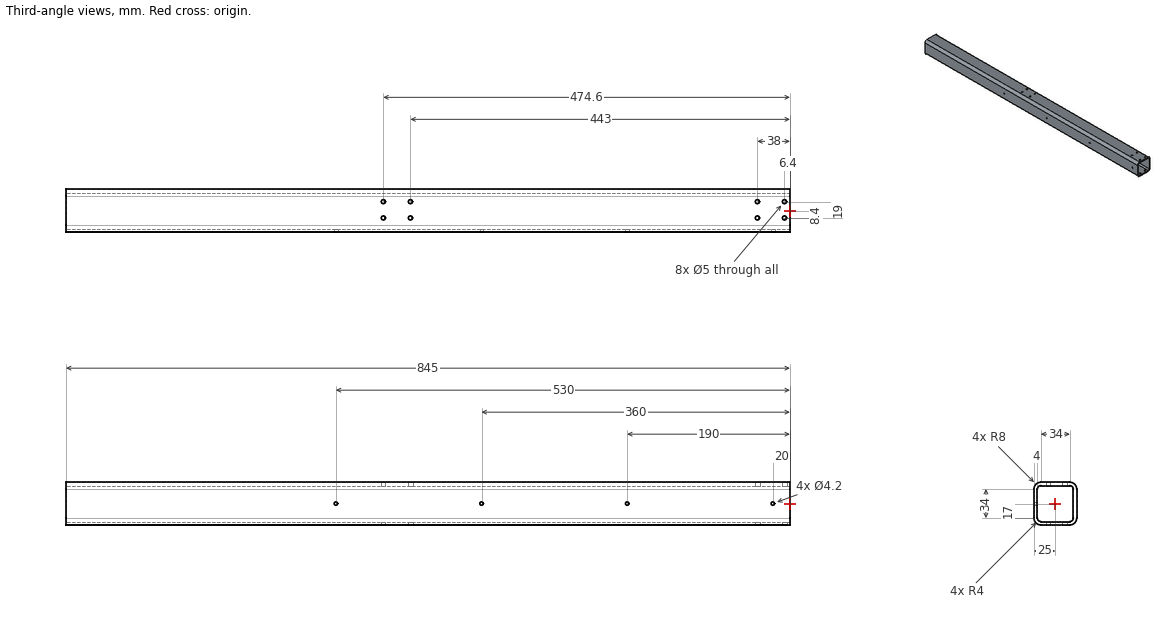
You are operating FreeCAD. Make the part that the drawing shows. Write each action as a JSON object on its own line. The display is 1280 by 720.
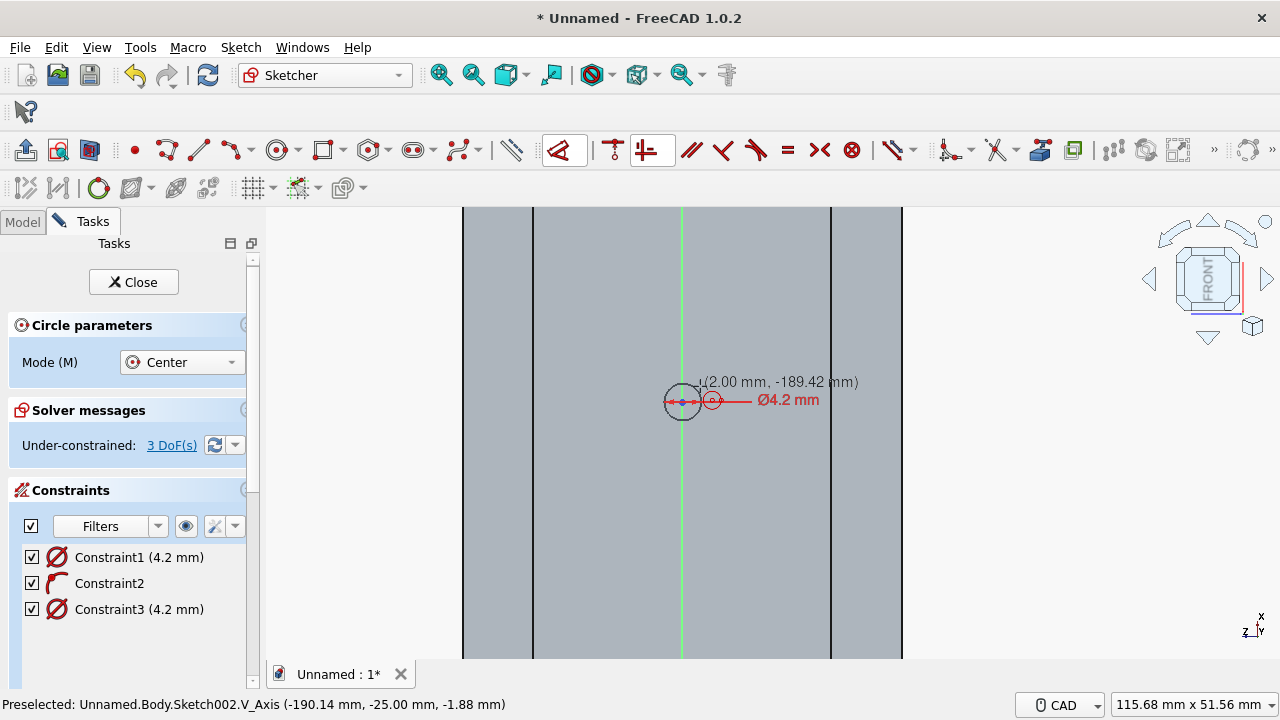
{"action": "scroll", "coordinate": [706, 392], "scroll_direction": "down", "scroll_amount": 14}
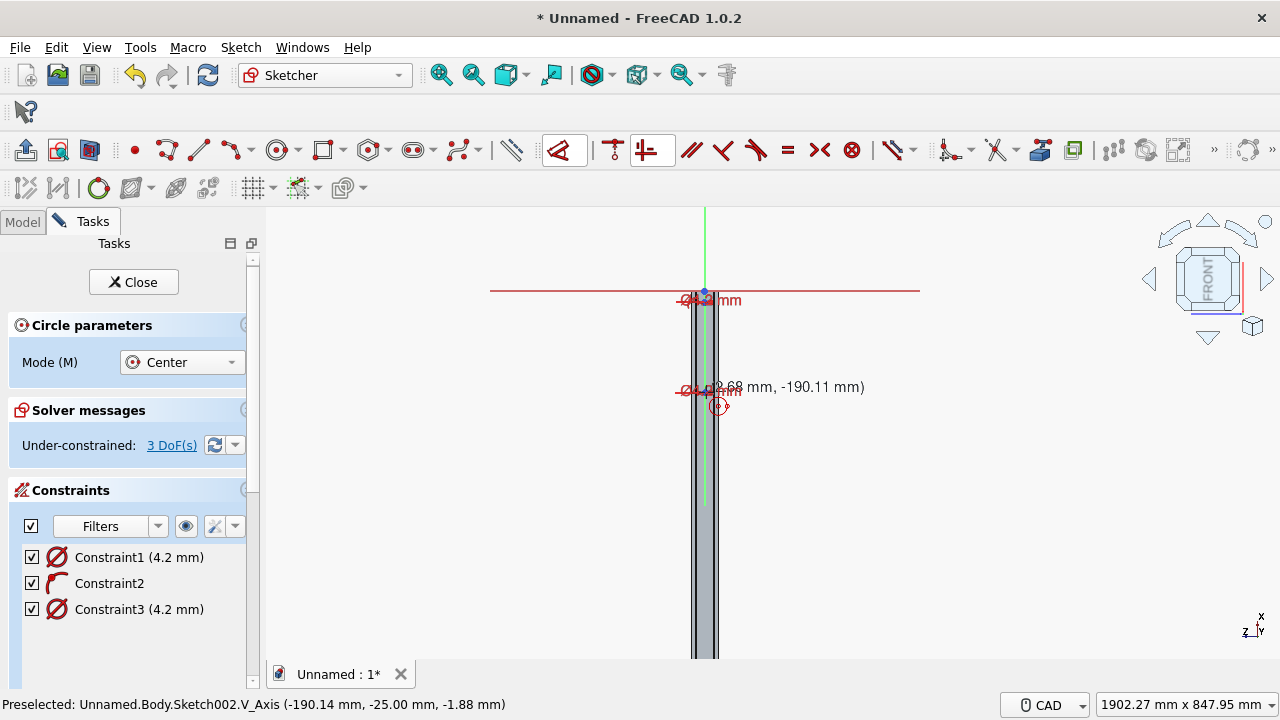
{"action": "scroll", "coordinate": [705, 483], "scroll_direction": "up", "scroll_amount": 16}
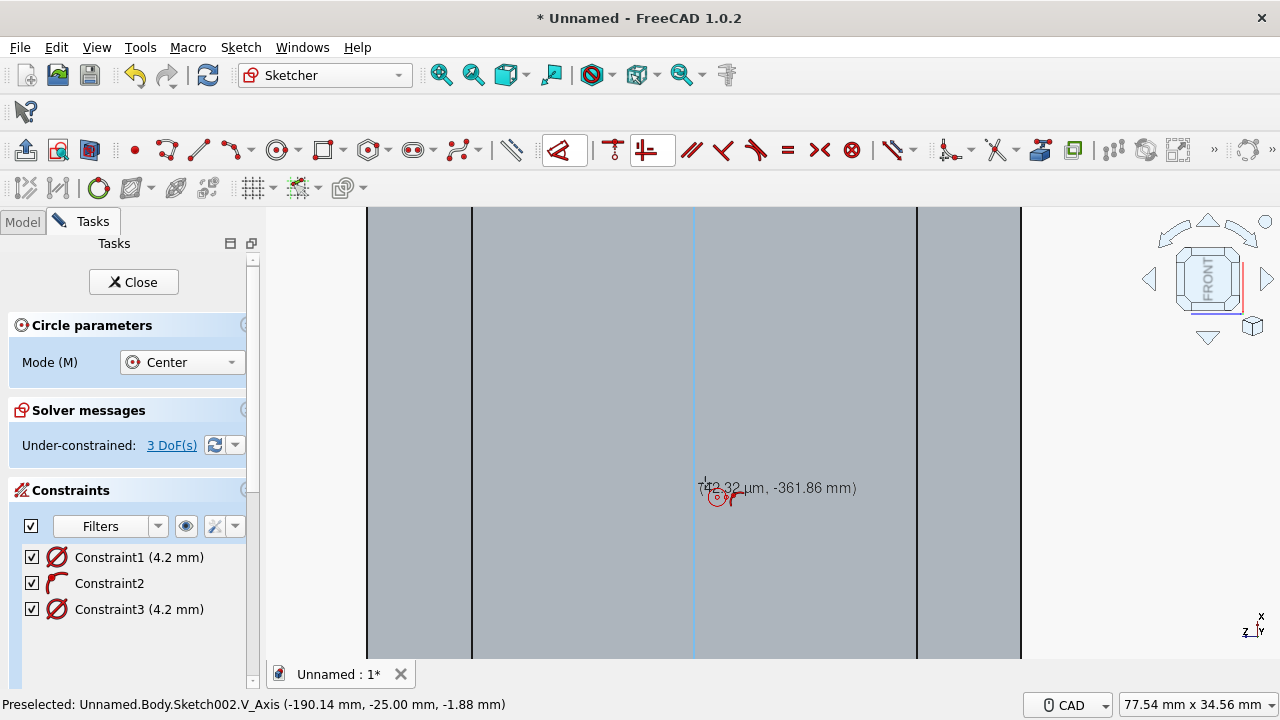
{"action": "scroll", "coordinate": [705, 484], "scroll_direction": "down", "scroll_amount": 16}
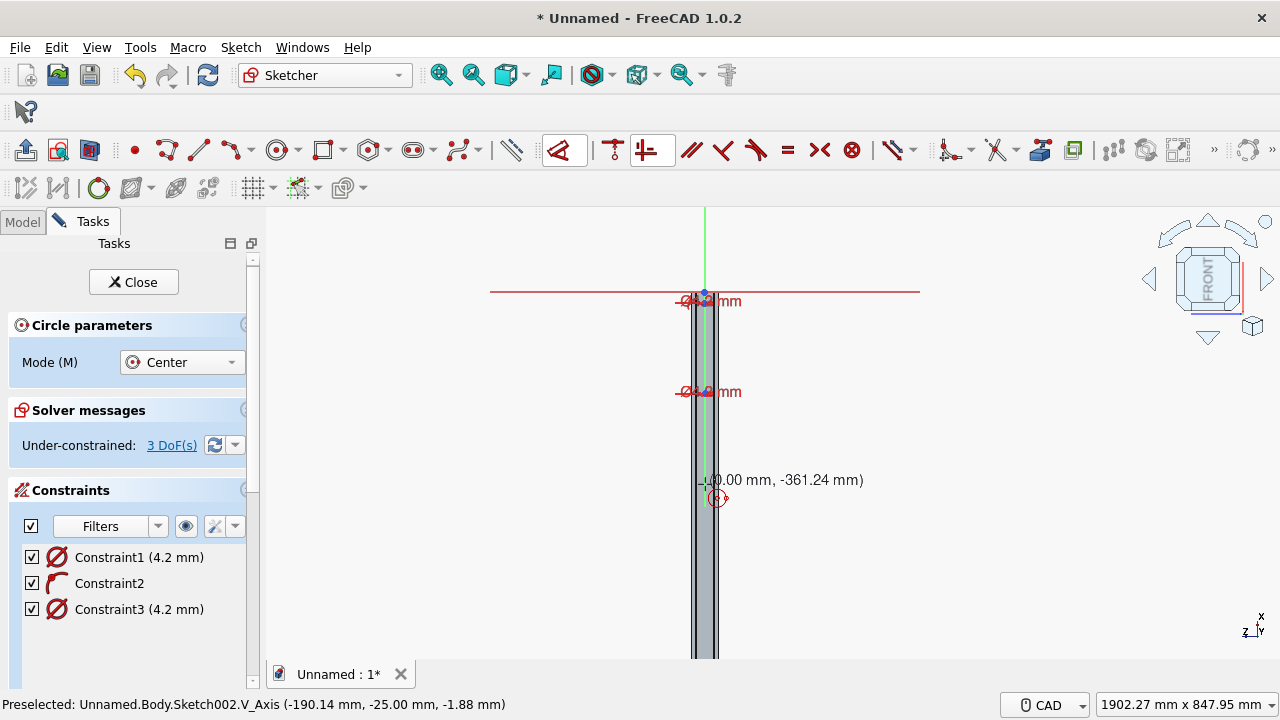
{"action": "left_click", "coordinate": [705, 484]}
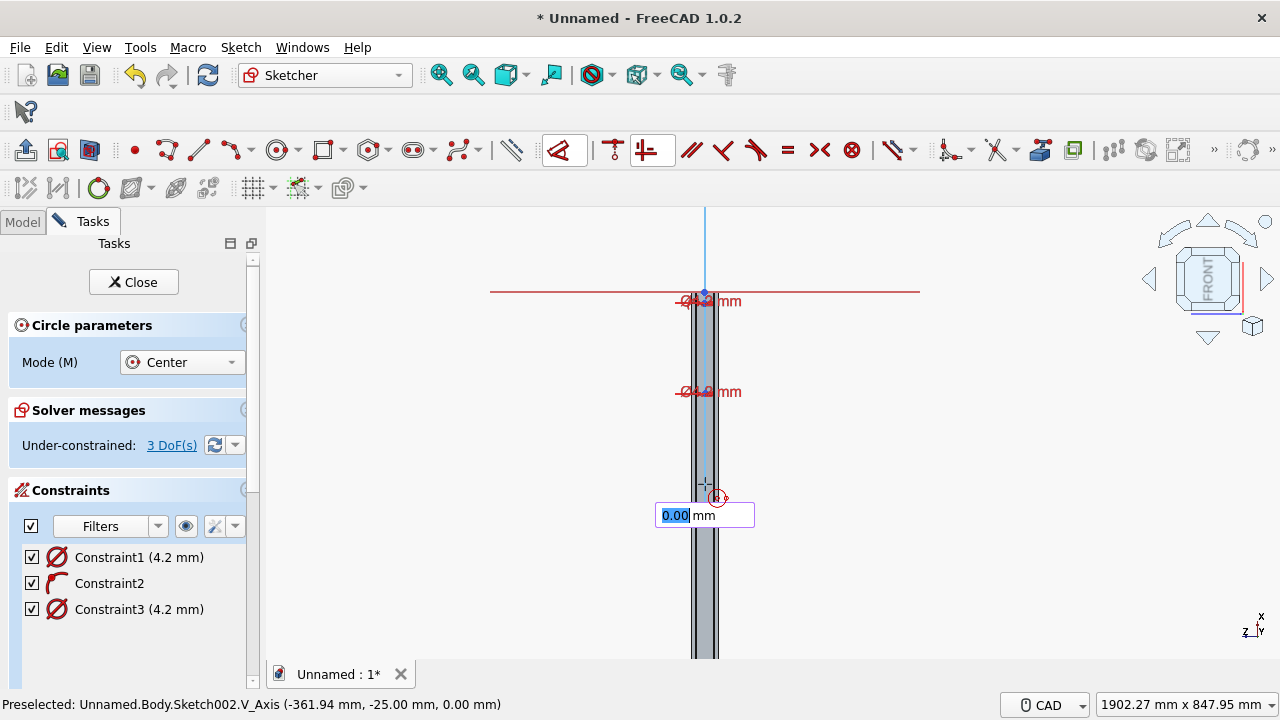
{"action": "scroll", "coordinate": [706, 484], "scroll_direction": "up", "scroll_amount": 14}
{"action": "mouse_move", "coordinate": [700, 468]}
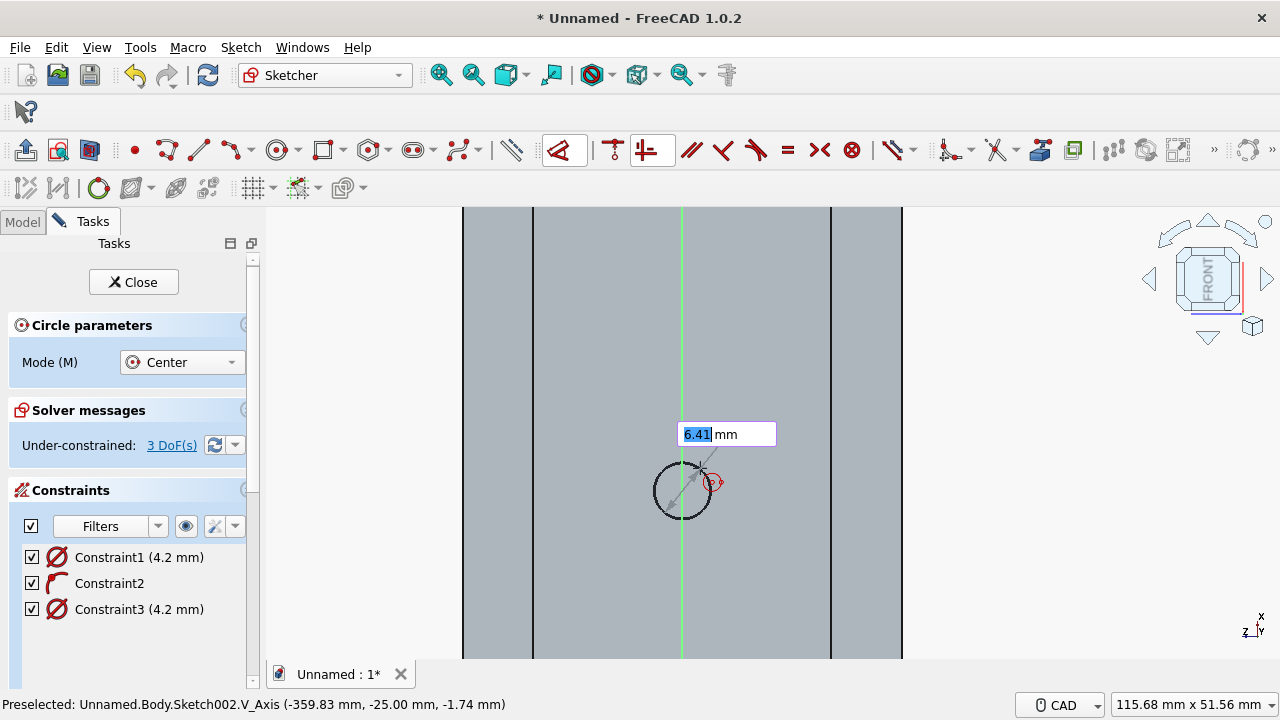
{"action": "type", "text": "4.2"}
{"action": "key", "text": "Return"}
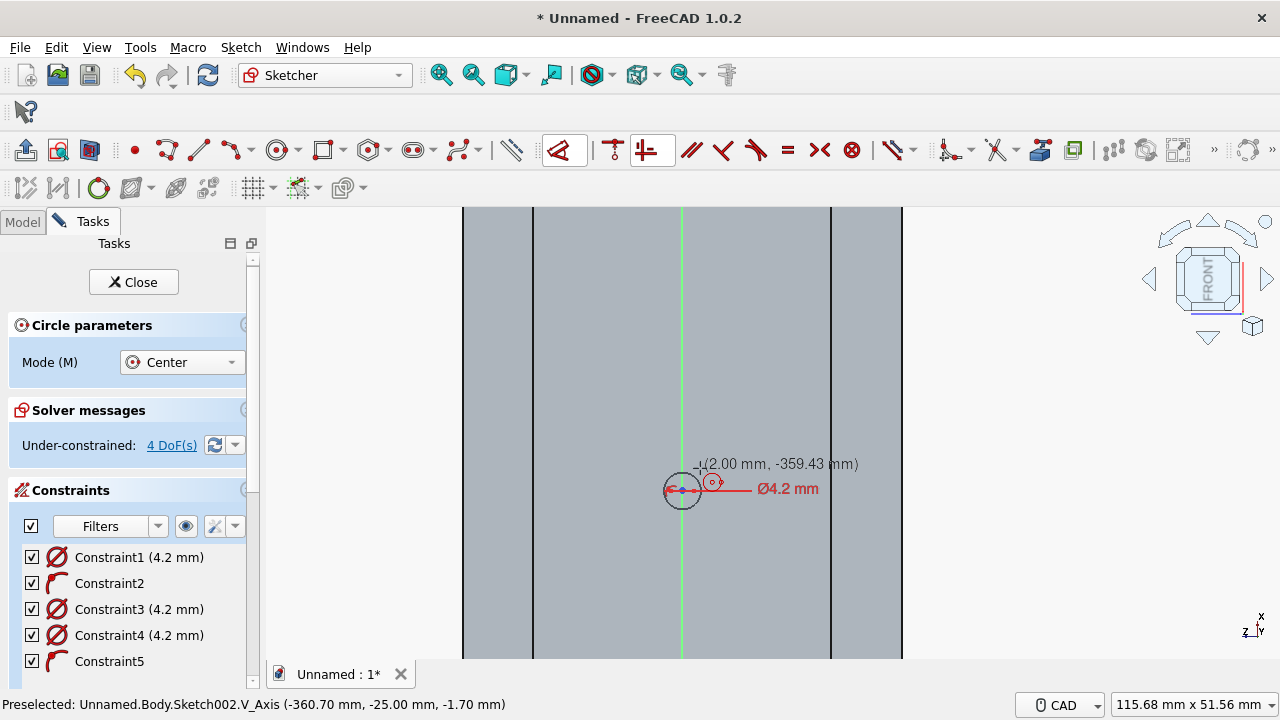
{"action": "scroll", "coordinate": [706, 484], "scroll_direction": "down", "scroll_amount": 14}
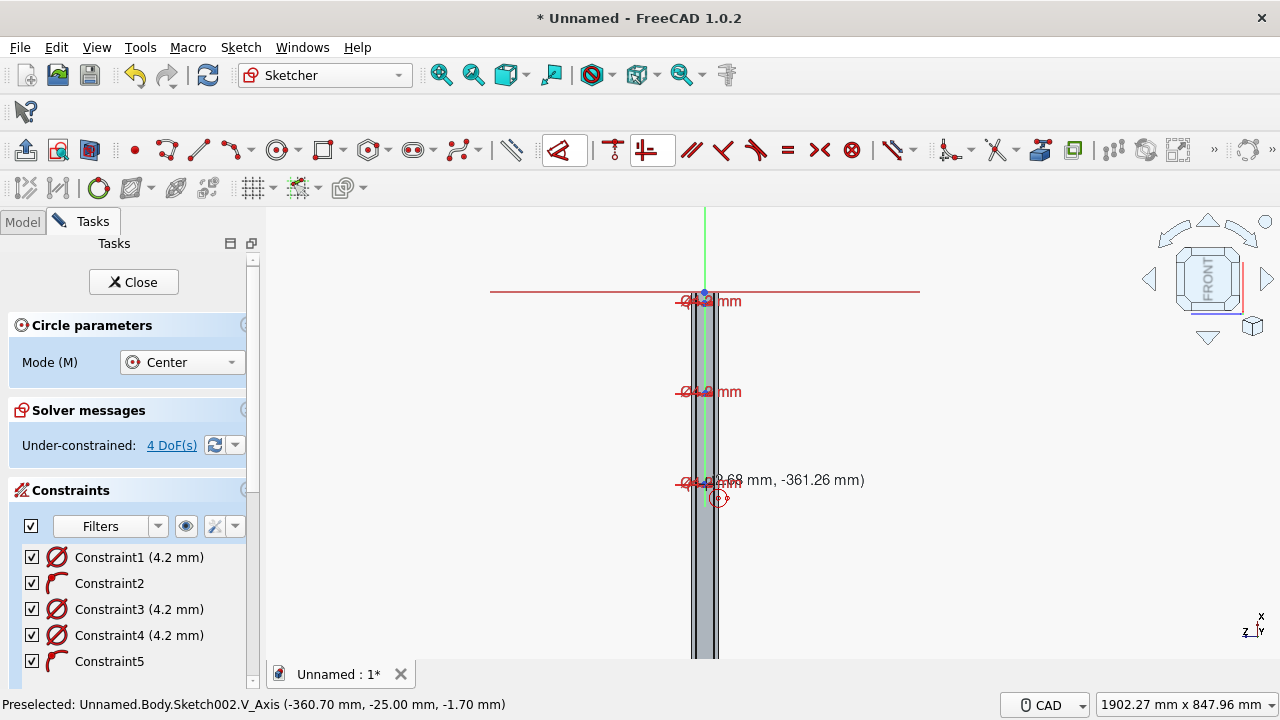
{"action": "scroll", "coordinate": [705, 575], "scroll_direction": "up", "scroll_amount": 16}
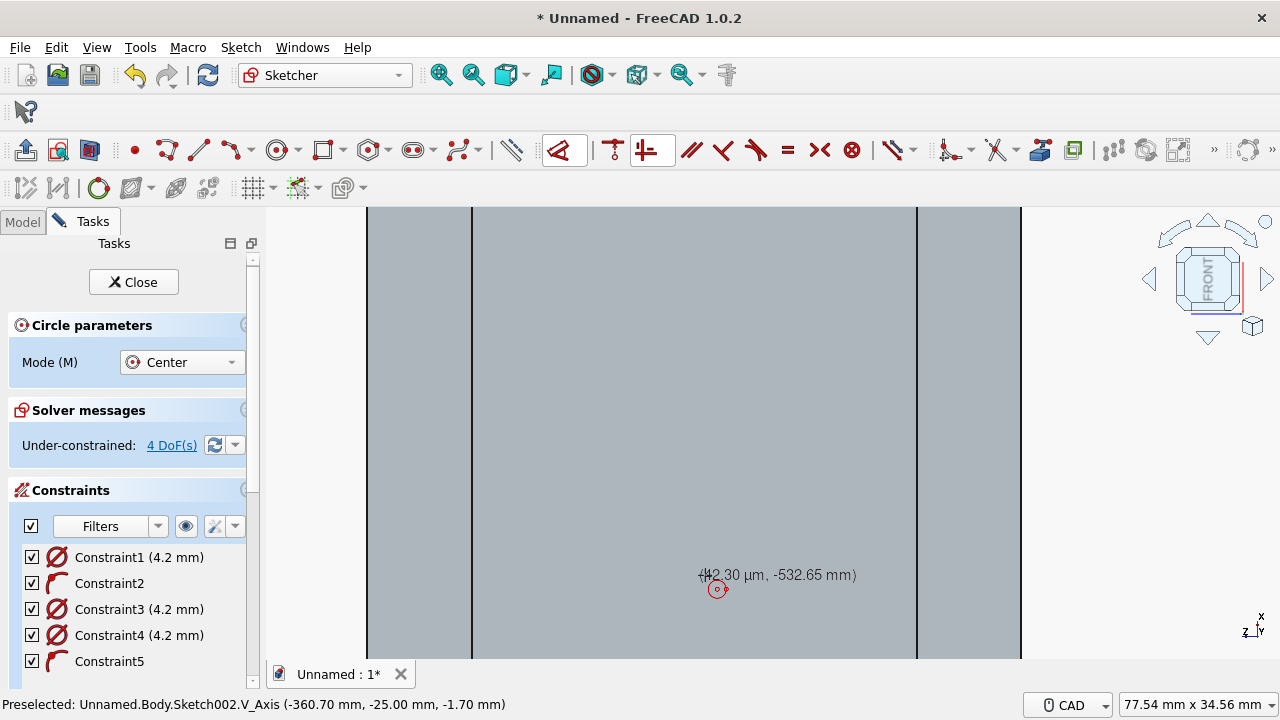
{"action": "scroll", "coordinate": [705, 575], "scroll_direction": "down", "scroll_amount": 16}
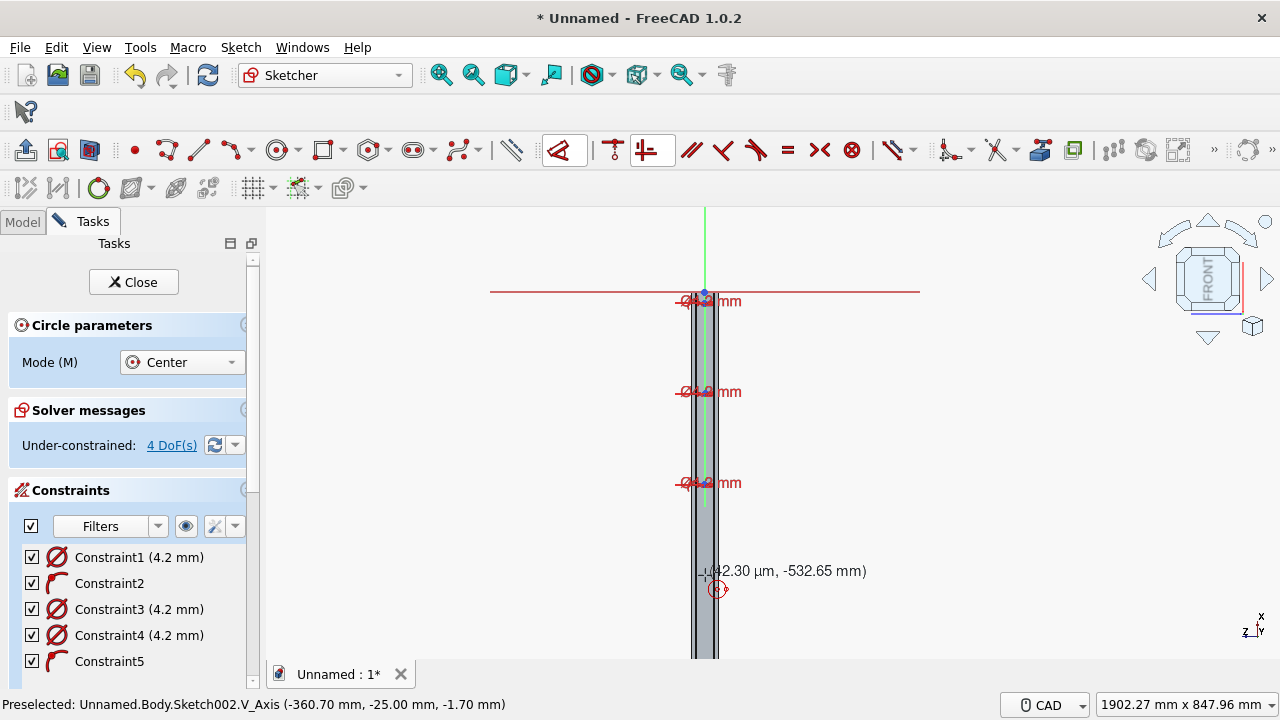
{"action": "left_click", "coordinate": [705, 575]}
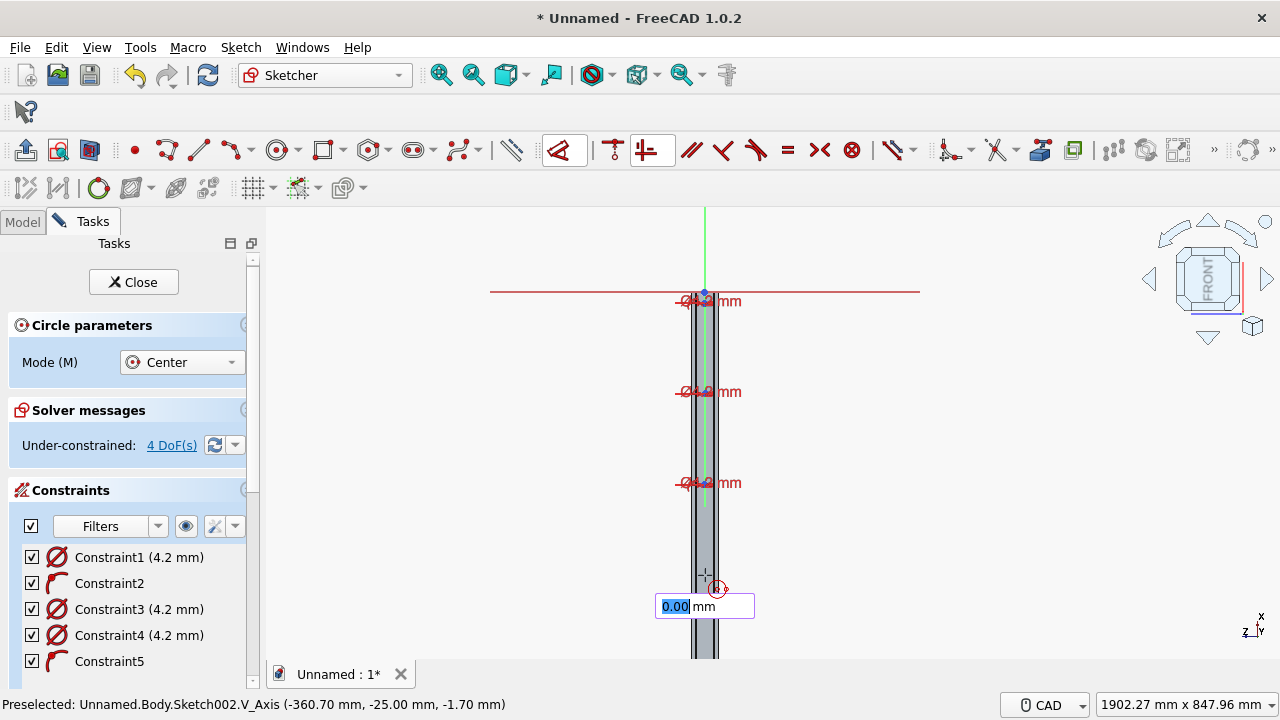
{"action": "scroll", "coordinate": [706, 574], "scroll_direction": "up", "scroll_amount": 14}
{"action": "mouse_move", "coordinate": [700, 565]}